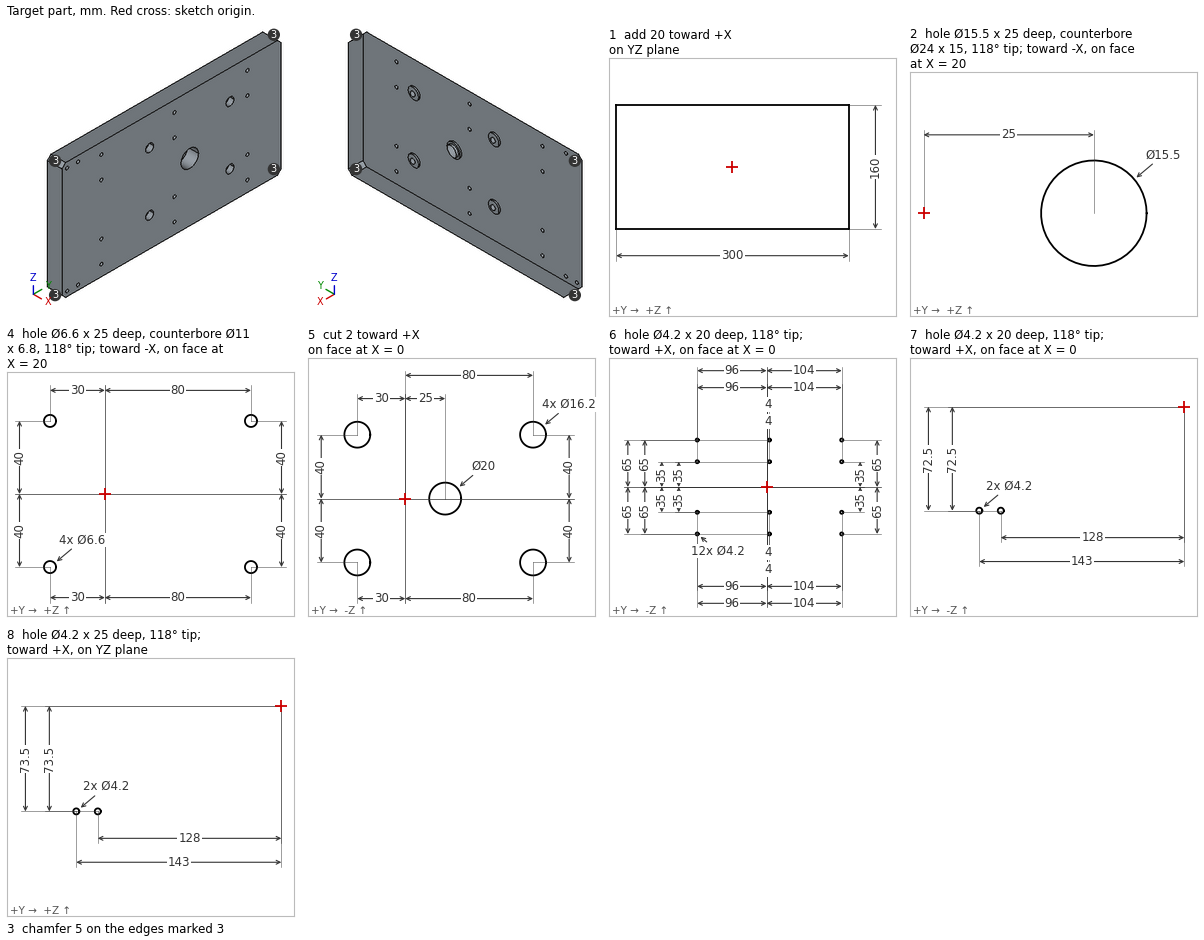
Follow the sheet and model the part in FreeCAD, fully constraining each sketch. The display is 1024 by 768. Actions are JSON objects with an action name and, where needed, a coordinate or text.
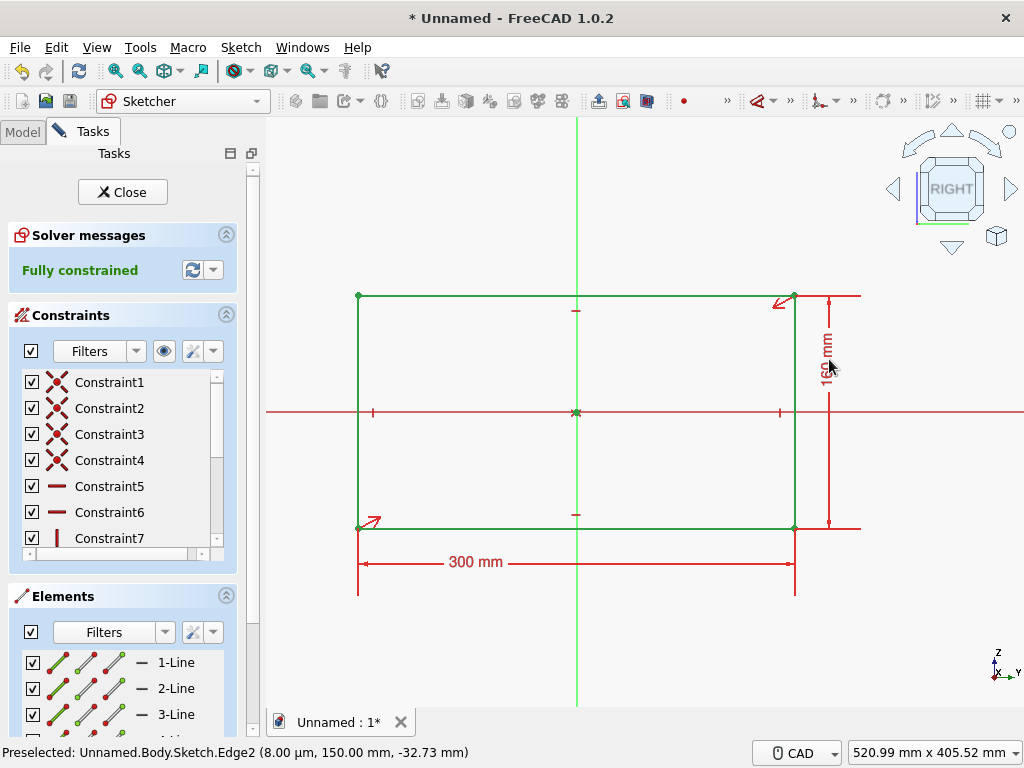
{"action": "left_click", "coordinate": [123, 192]}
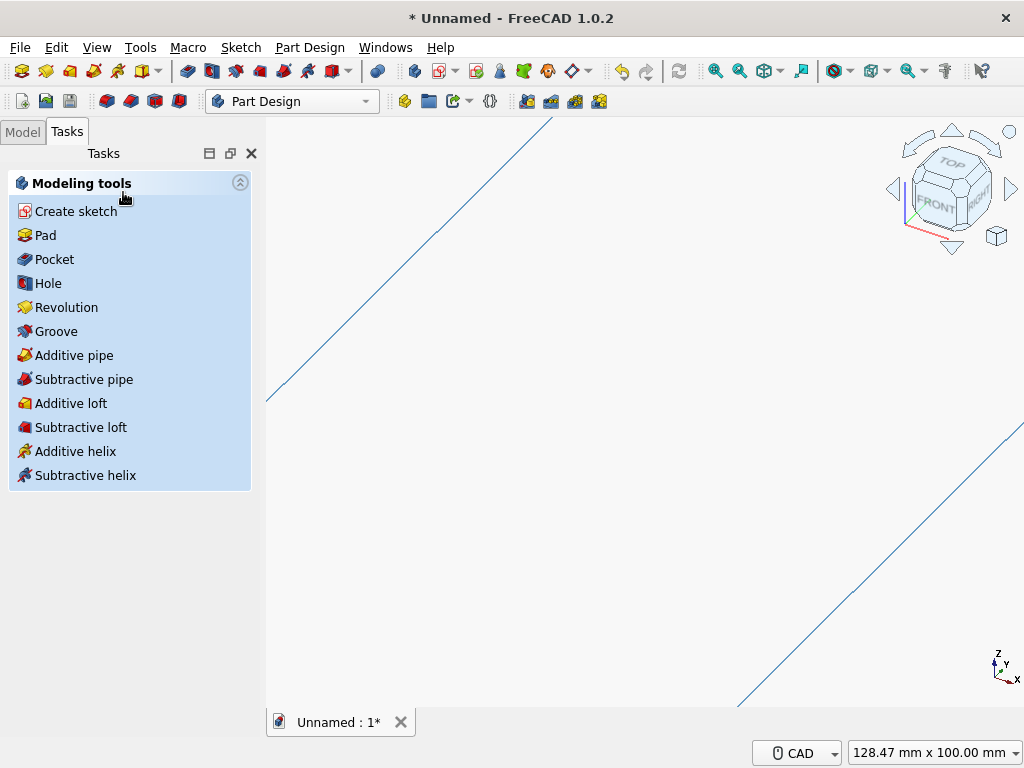
{"action": "left_click", "coordinate": [22, 72]}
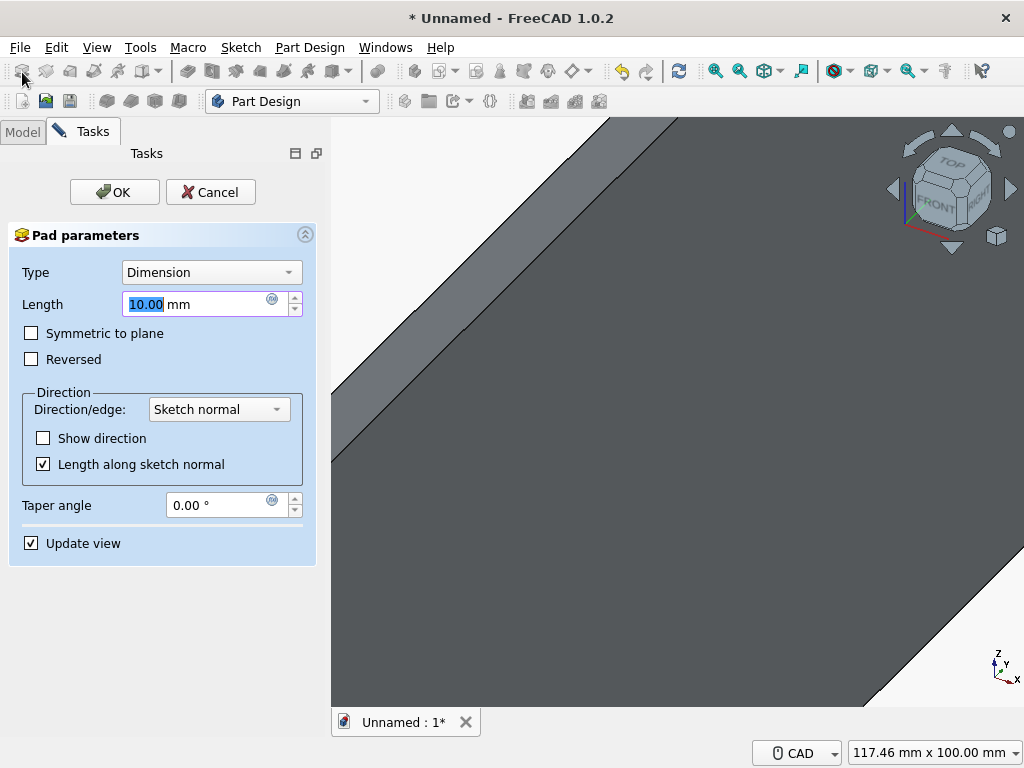
{"action": "type", "text": "20"}
{"action": "key", "text": "Tab"}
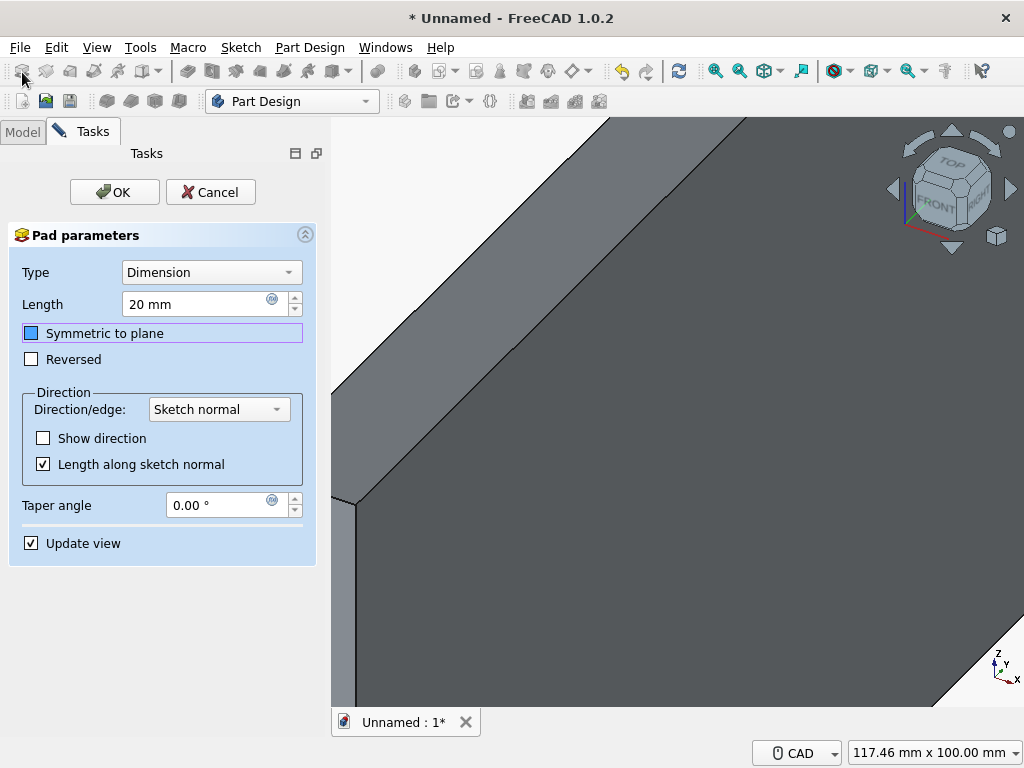
{"action": "left_click", "coordinate": [115, 192]}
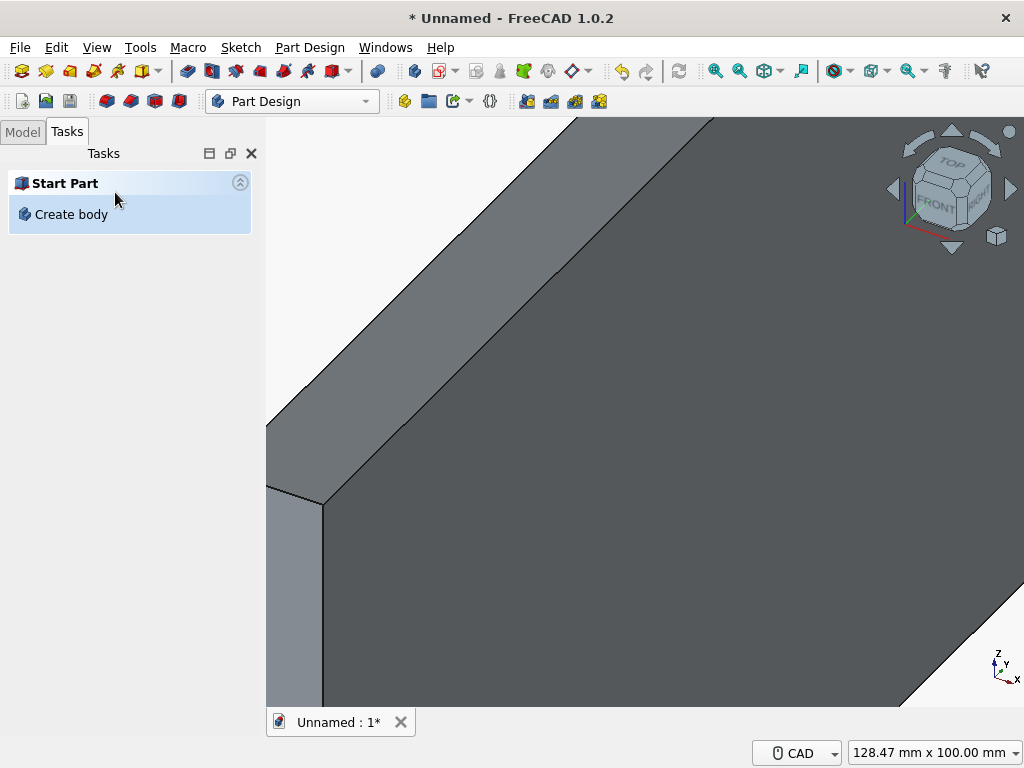
{"action": "key", "text": "v f"}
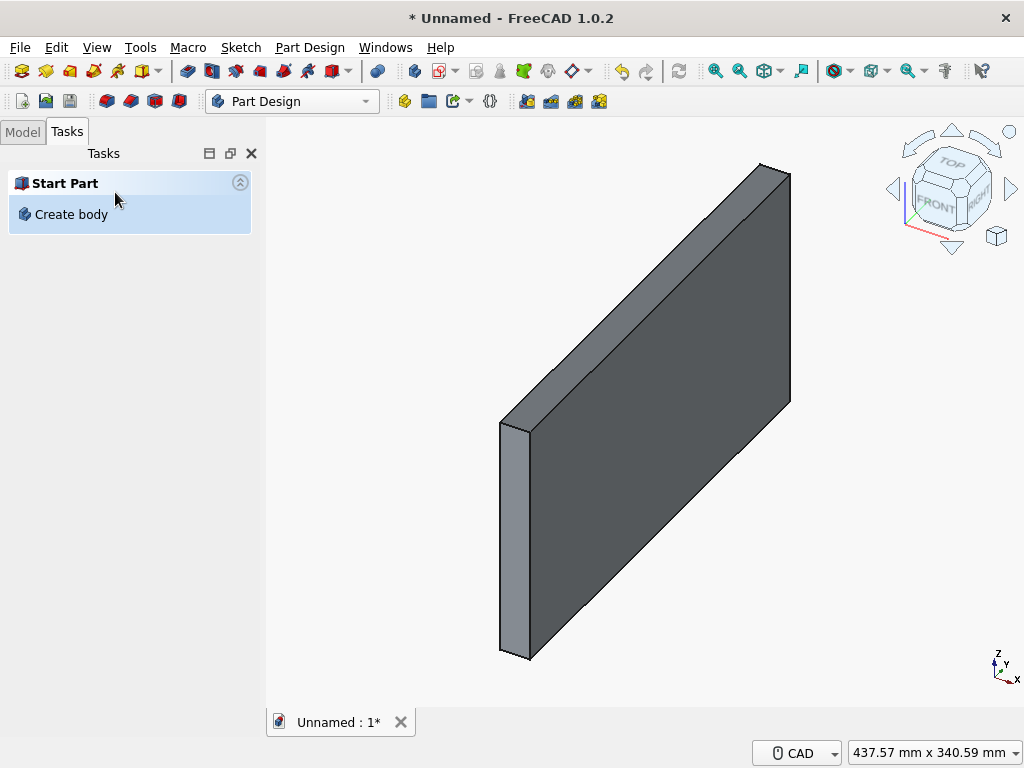
{"action": "left_click", "coordinate": [697, 379]}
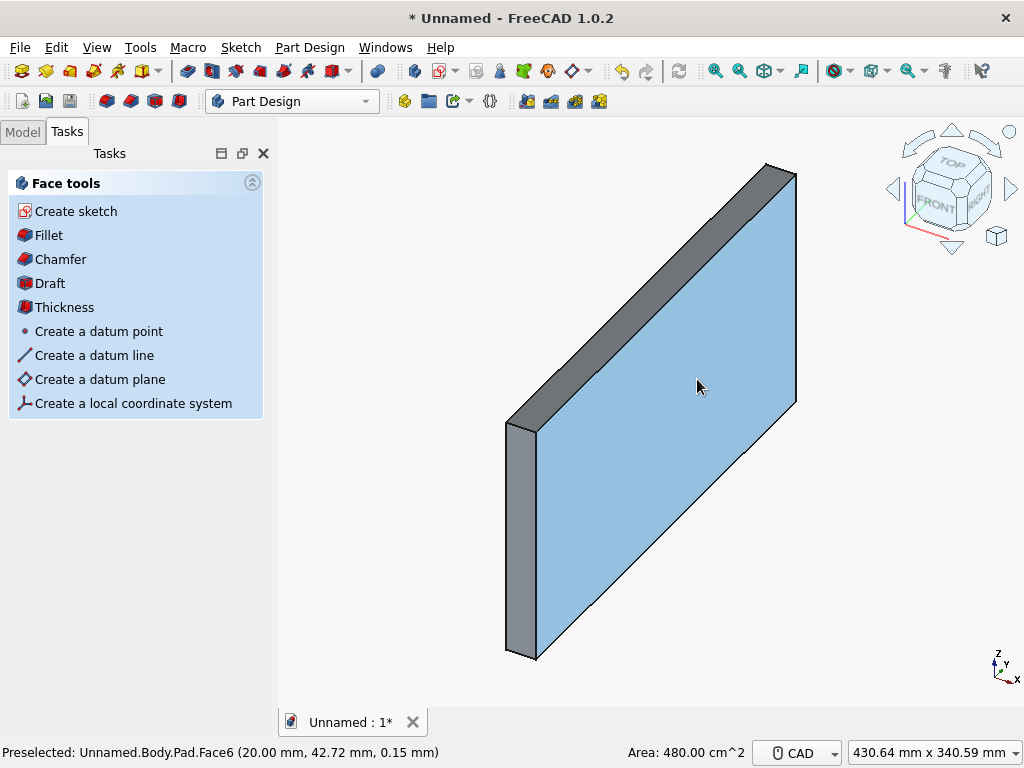
{"action": "left_click", "coordinate": [440, 72]}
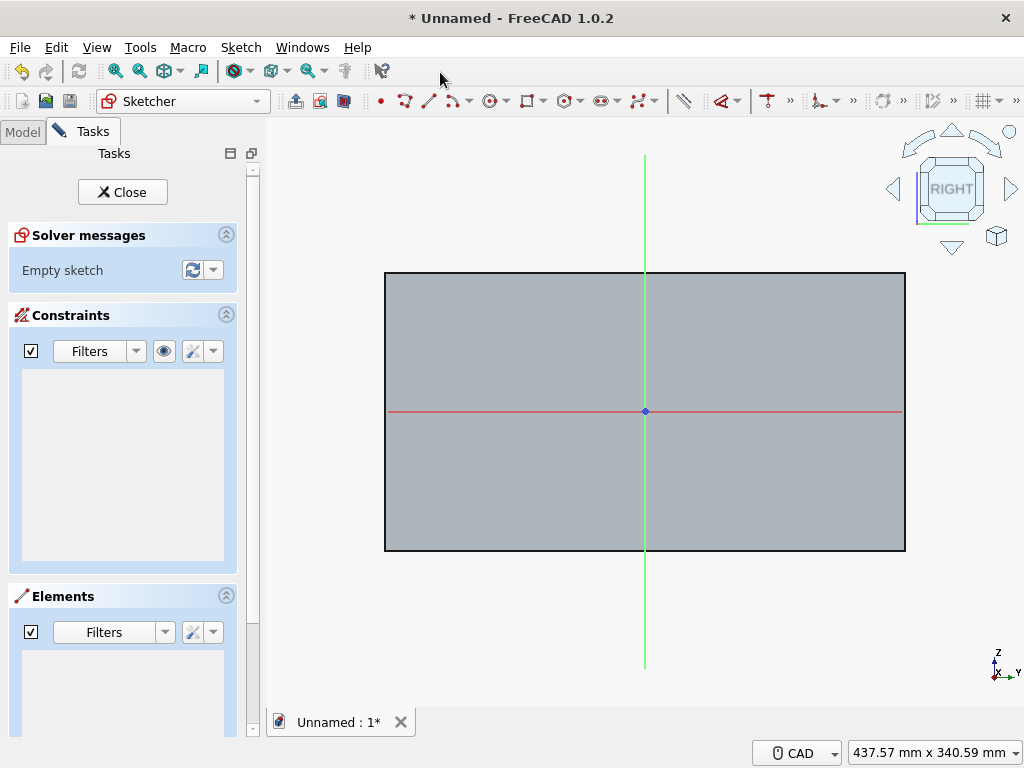
{"action": "scroll", "coordinate": [689, 412], "scroll_direction": "up", "scroll_amount": 10}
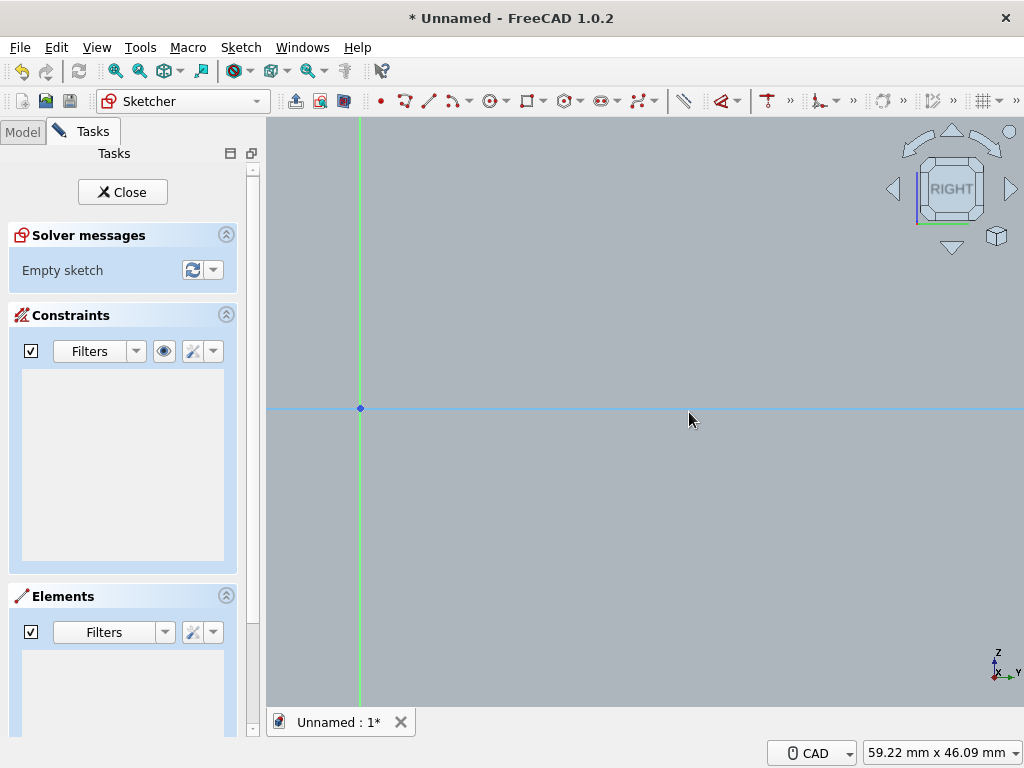
{"action": "left_click", "coordinate": [490, 102]}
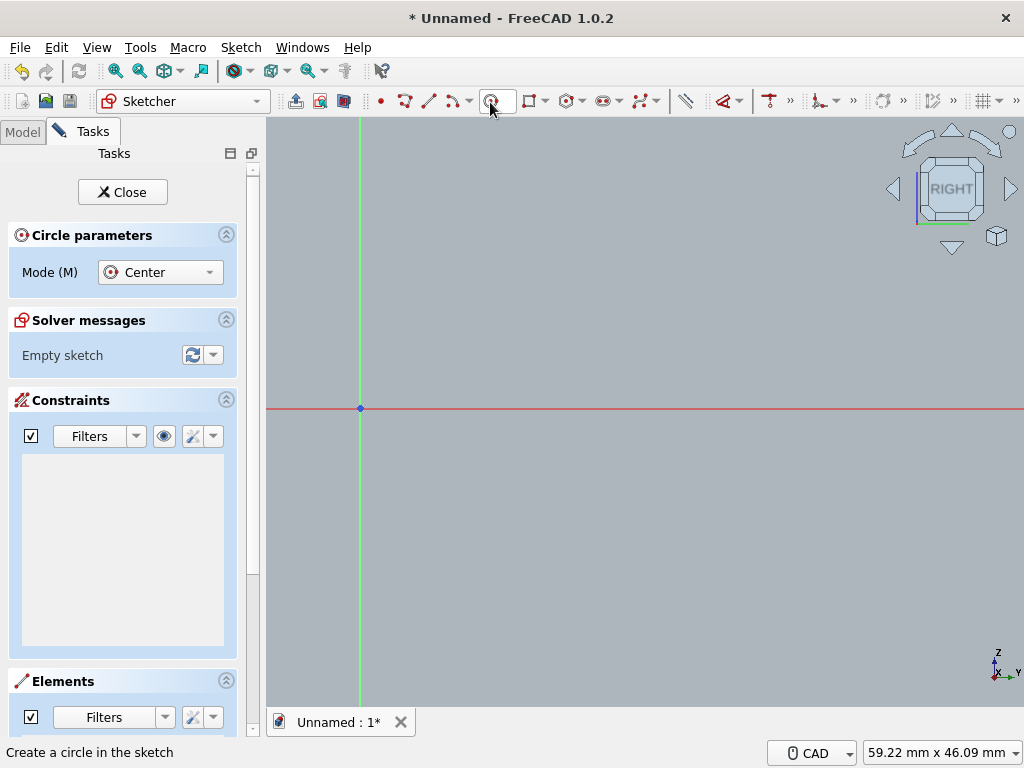
{"action": "left_click", "coordinate": [680, 409]}
{"action": "left_click", "coordinate": [750, 339]}
{"action": "key", "text": "Escape"}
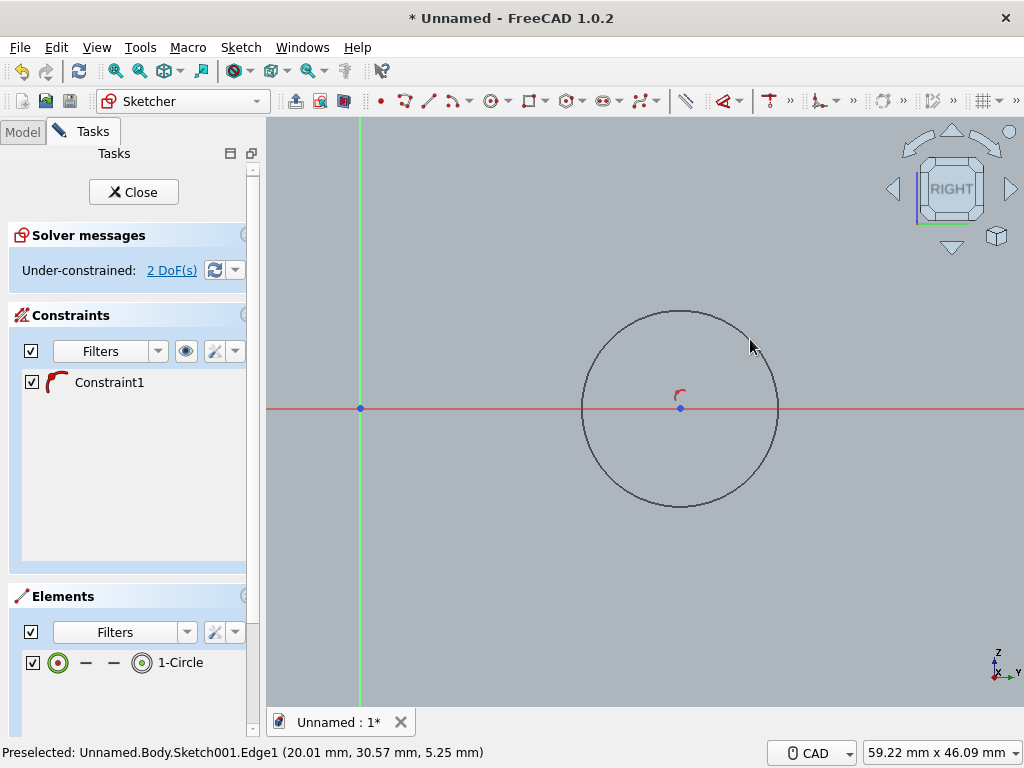
{"action": "key", "text": "d"}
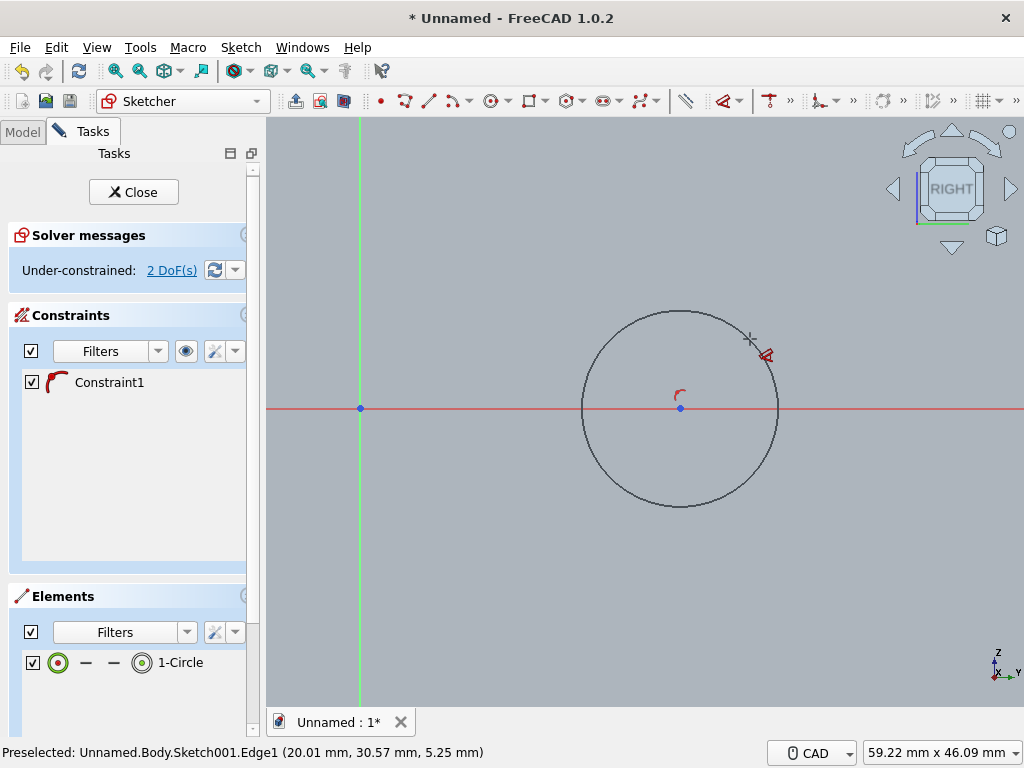
{"action": "left_click", "coordinate": [749, 339]}
{"action": "left_click", "coordinate": [771, 316]}